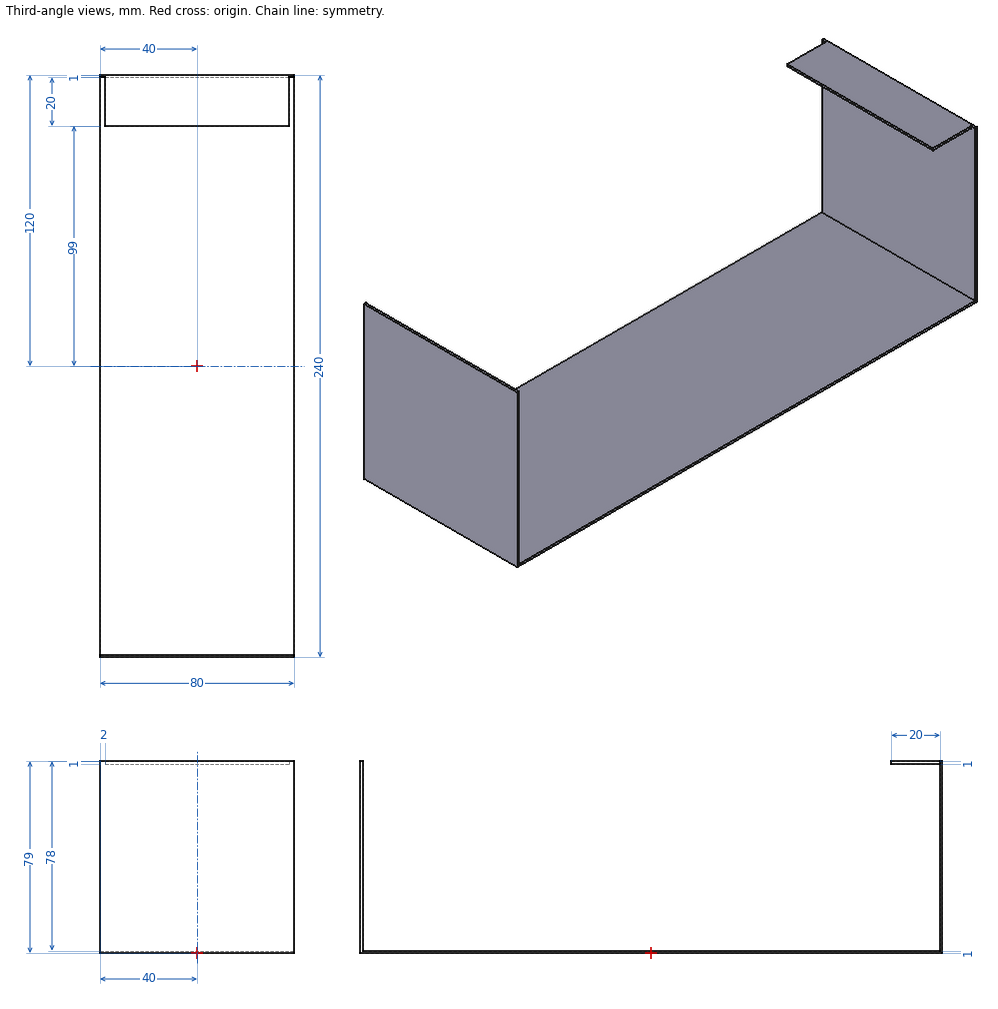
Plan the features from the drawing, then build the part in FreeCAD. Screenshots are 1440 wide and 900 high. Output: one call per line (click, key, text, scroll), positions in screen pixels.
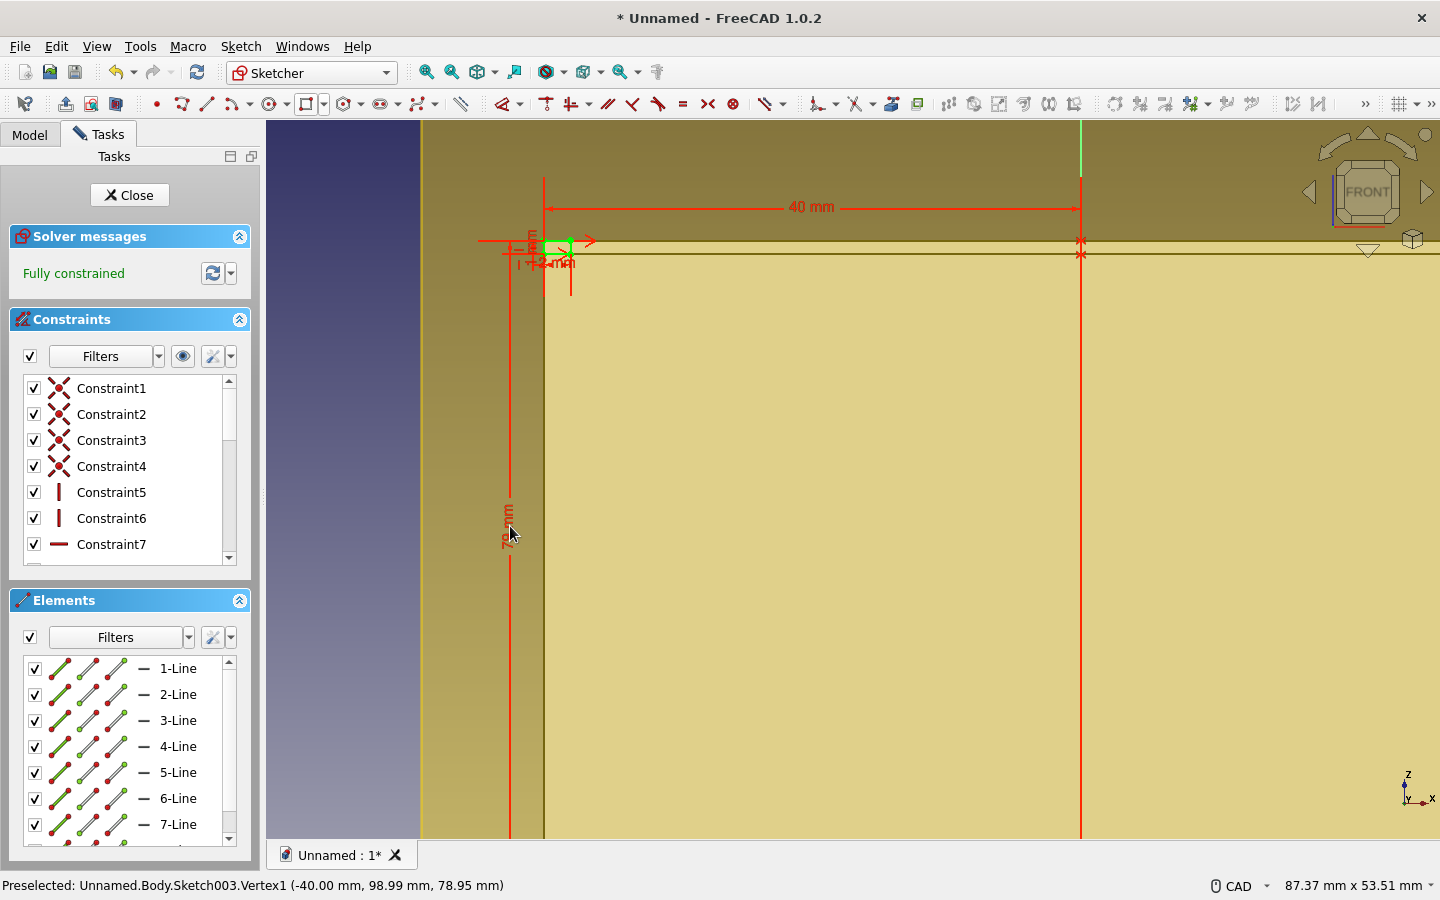
click(130, 195)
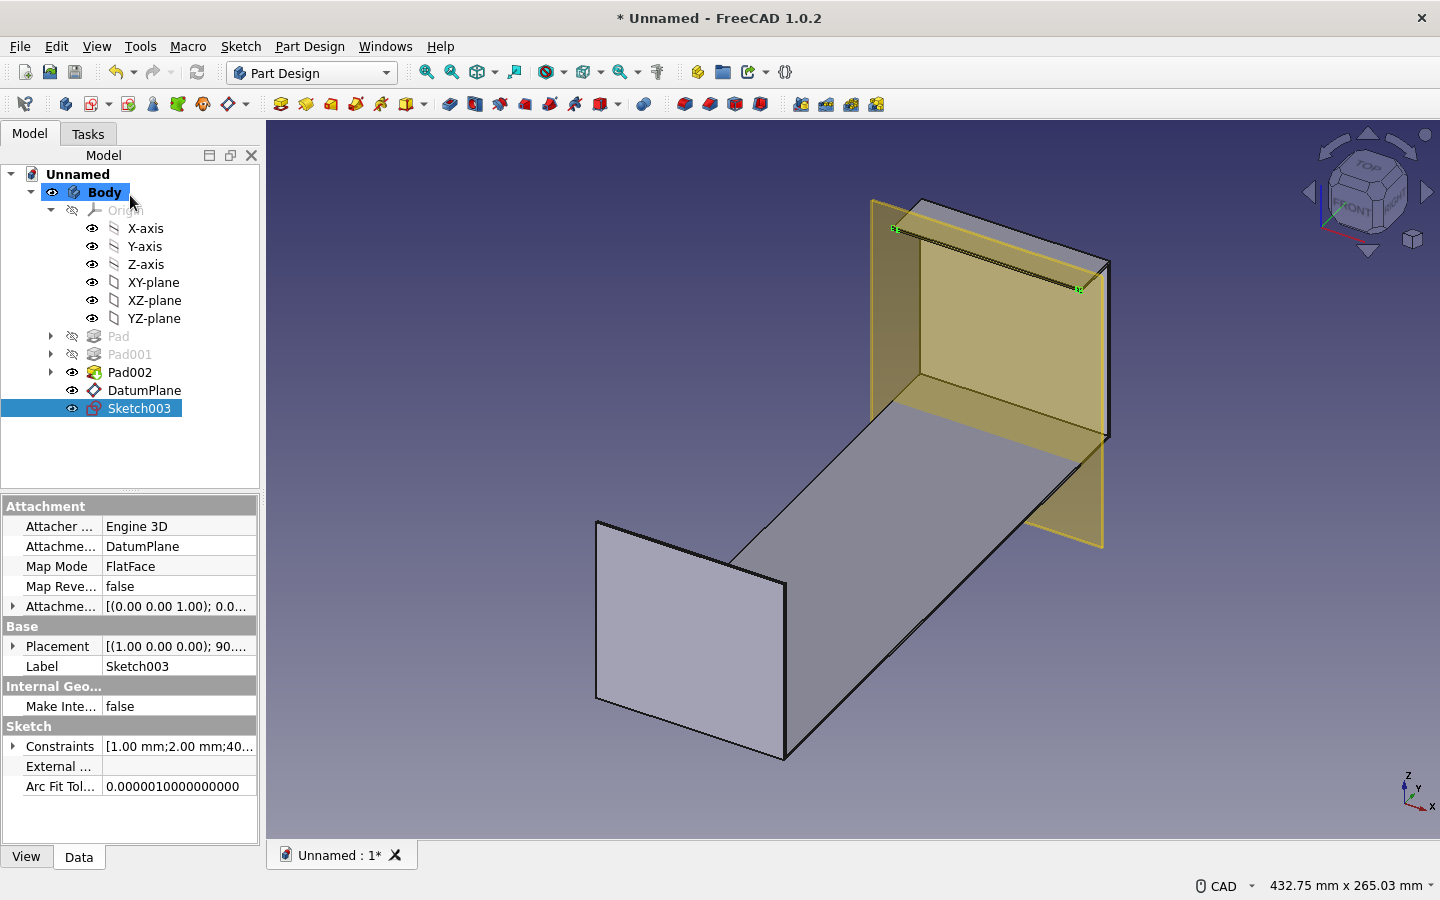
click(450, 104)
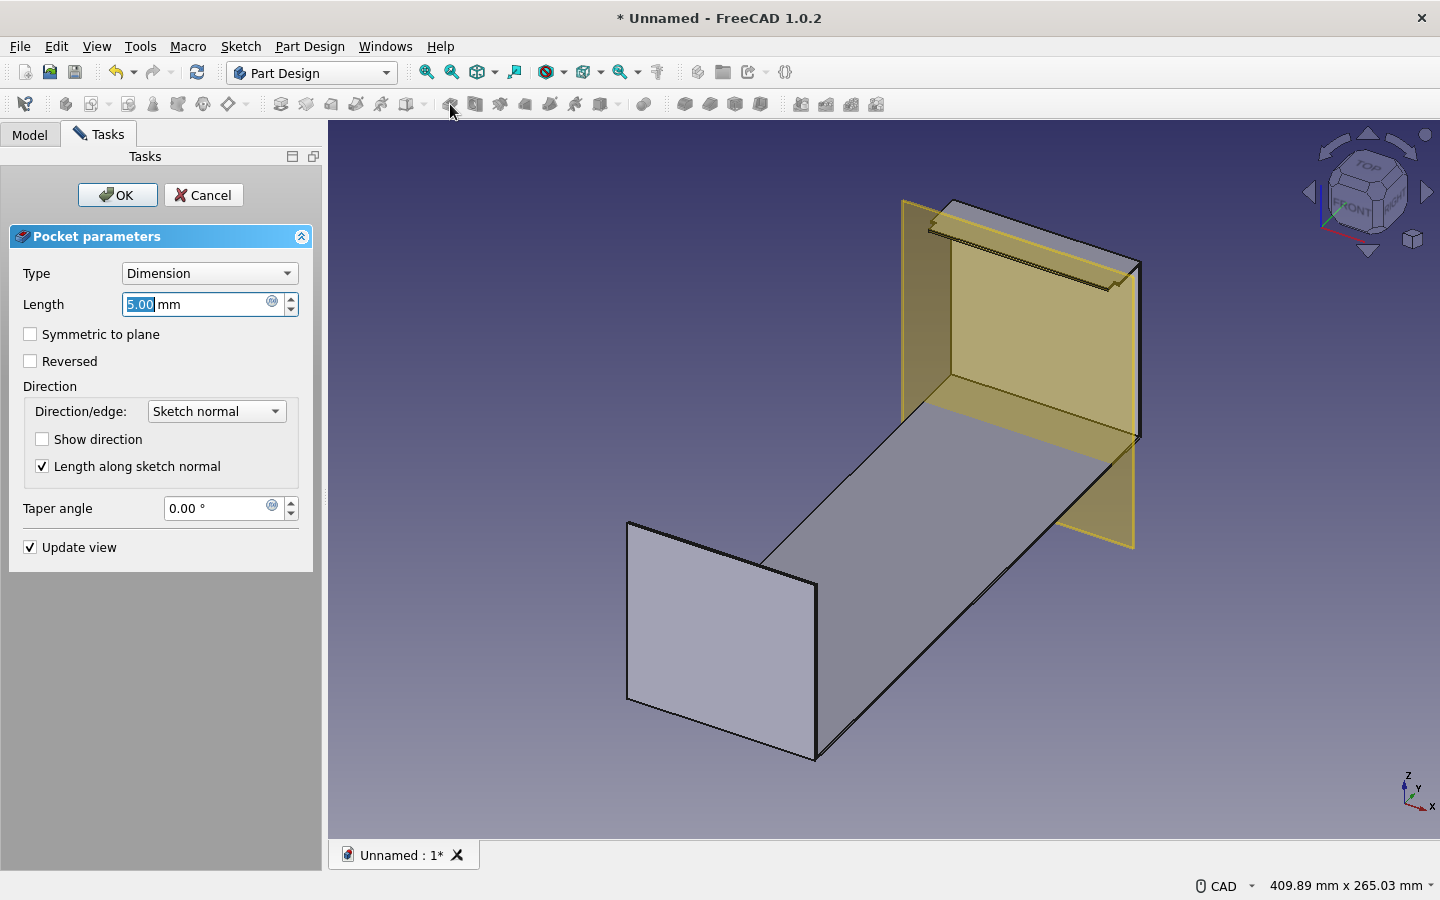
text(20)
key(Tab)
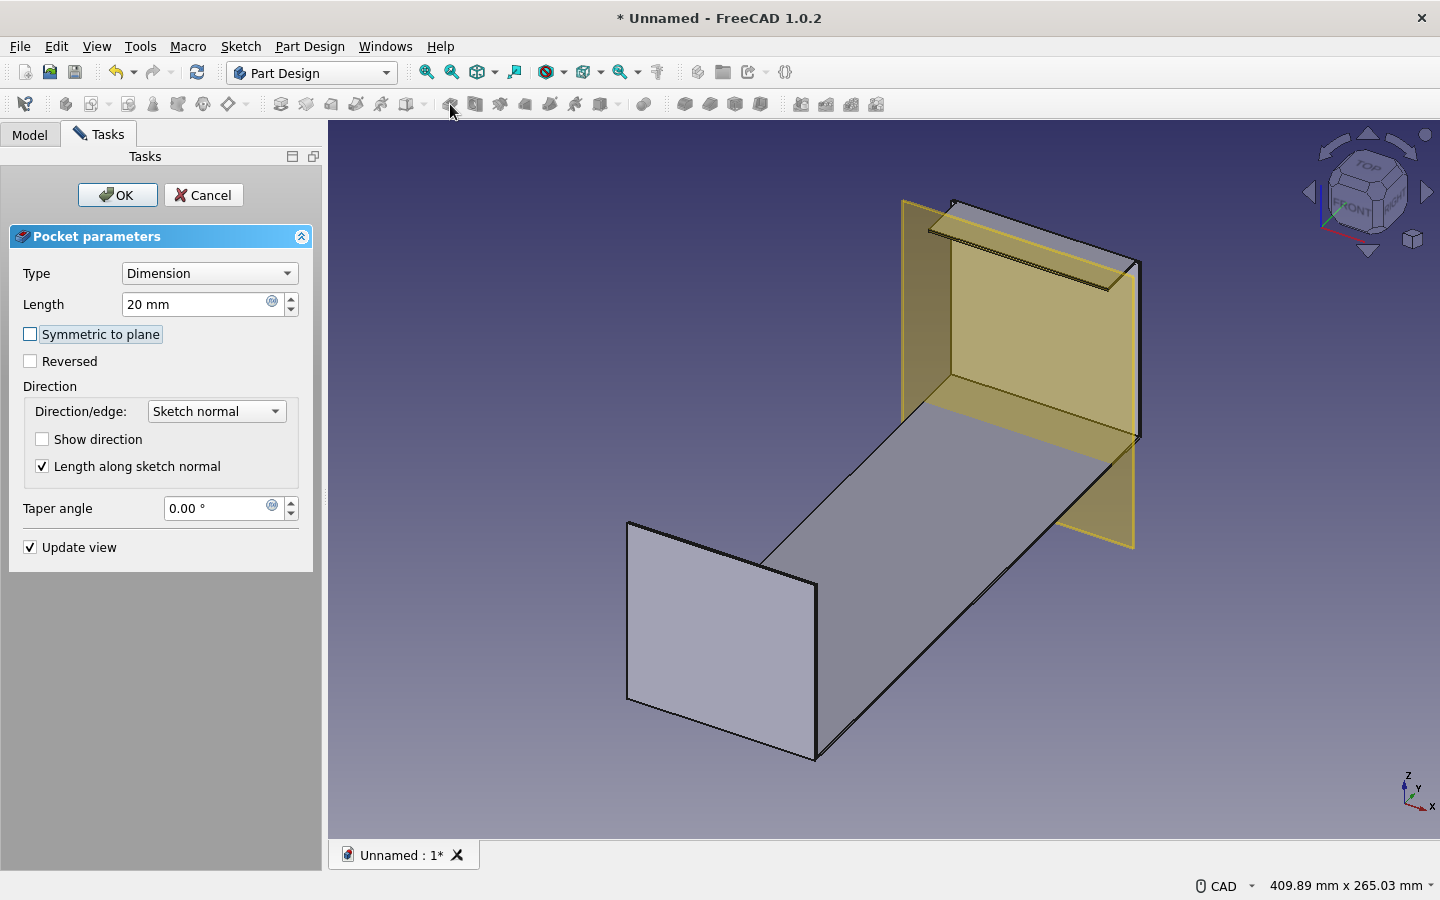
click(118, 195)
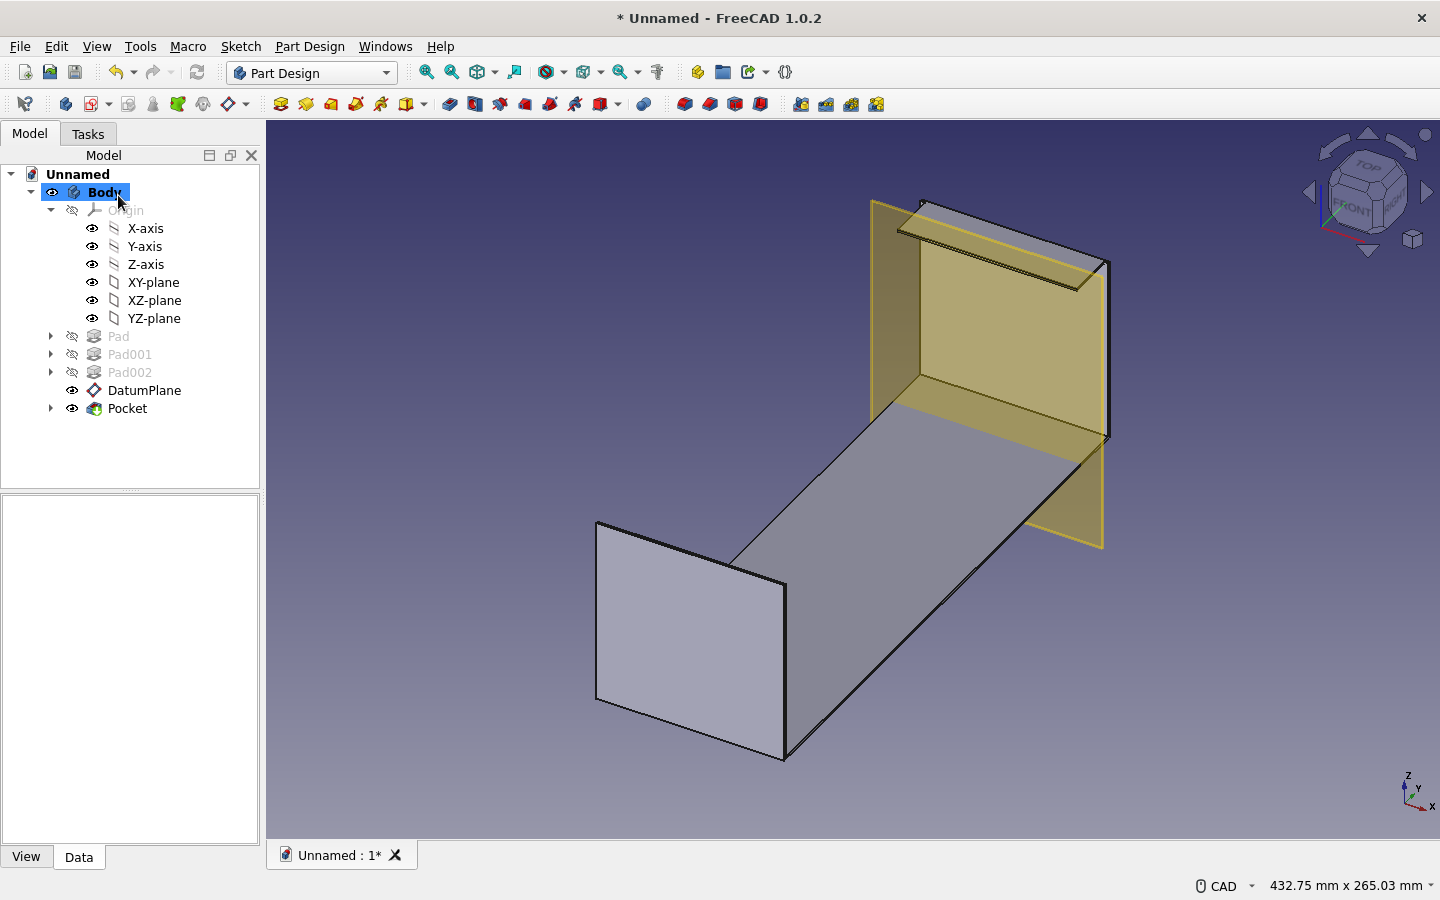
click(117, 390)
key(space)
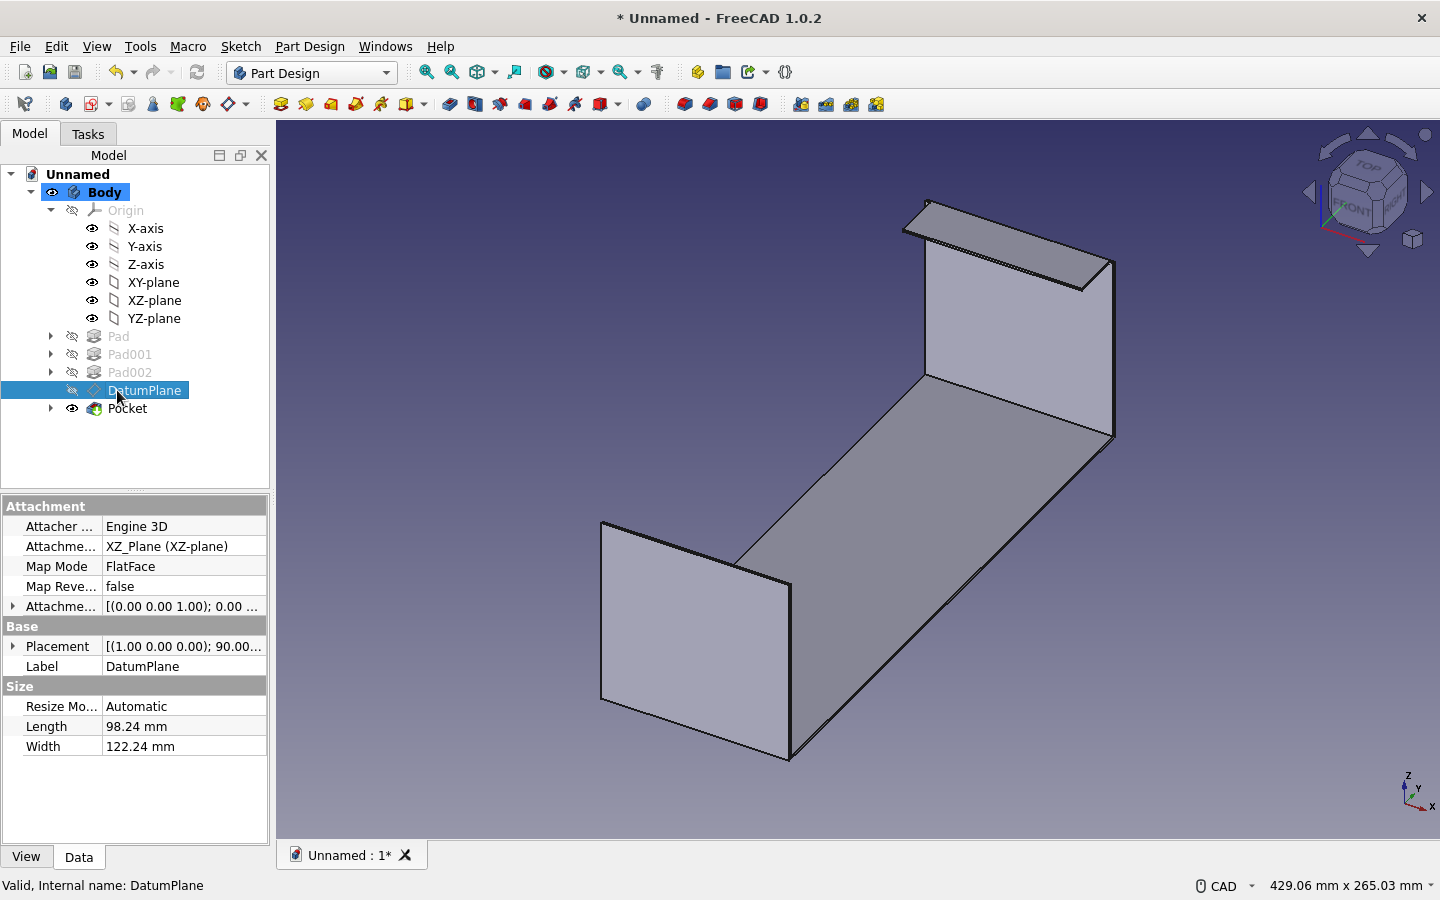
key(0)